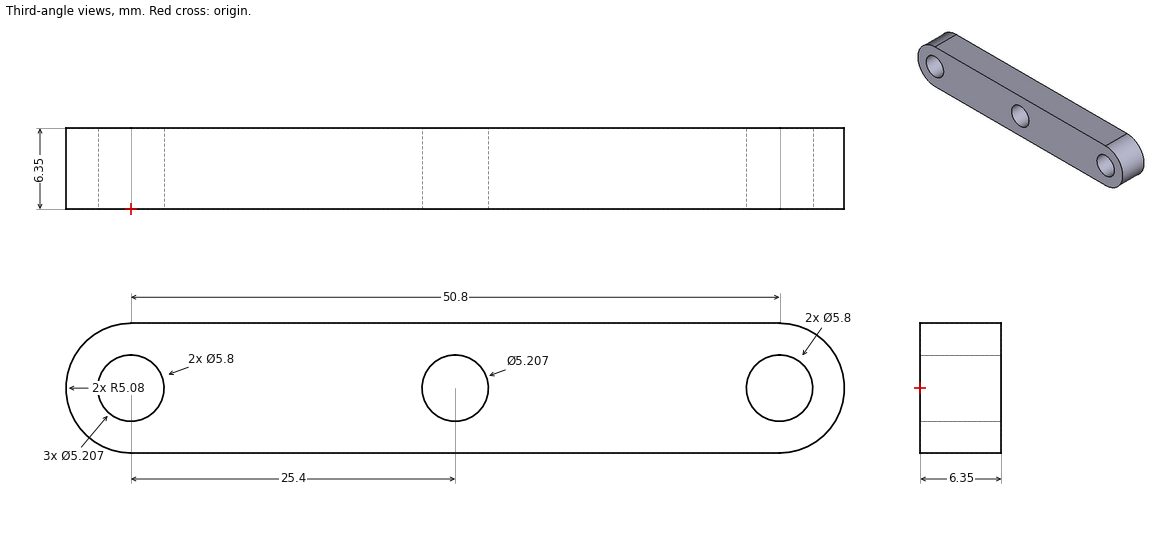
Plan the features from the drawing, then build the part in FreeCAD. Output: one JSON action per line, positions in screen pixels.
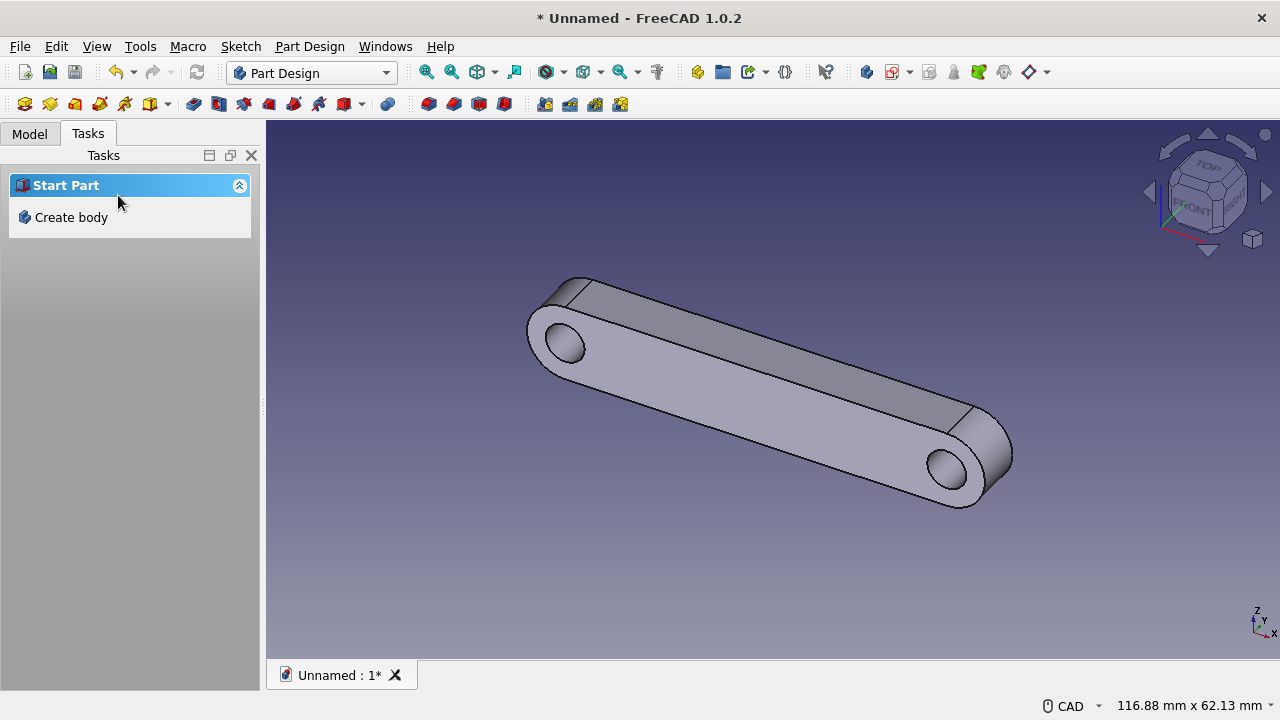
{"action": "key", "text": "4"}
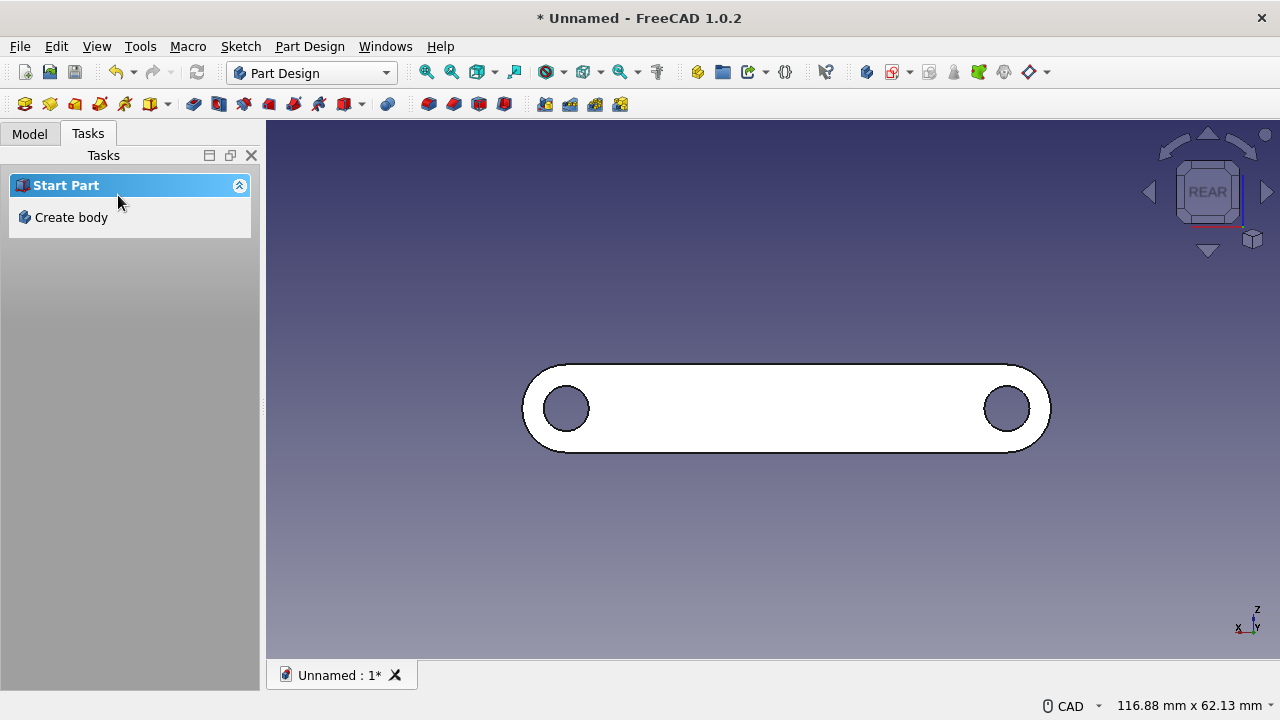
{"action": "left_click", "coordinate": [635, 408]}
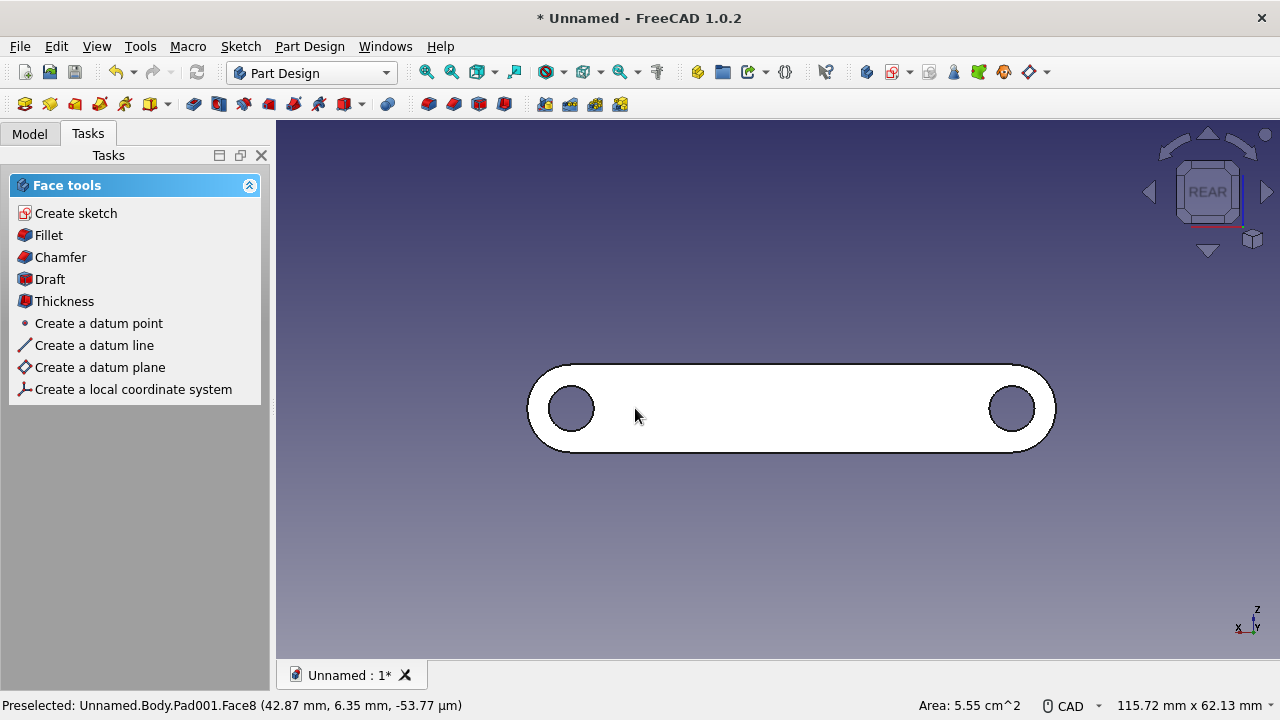
{"action": "left_click", "coordinate": [892, 72]}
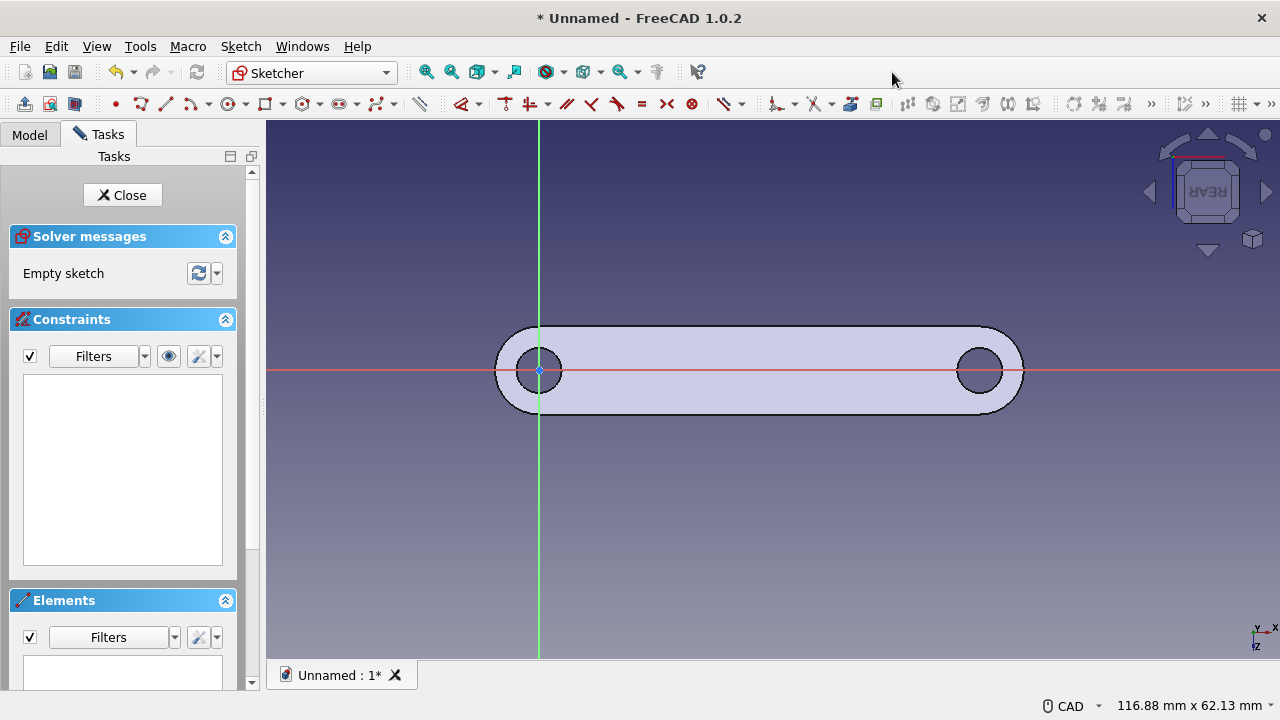
{"action": "scroll", "coordinate": [768, 367], "scroll_direction": "up", "scroll_amount": 10}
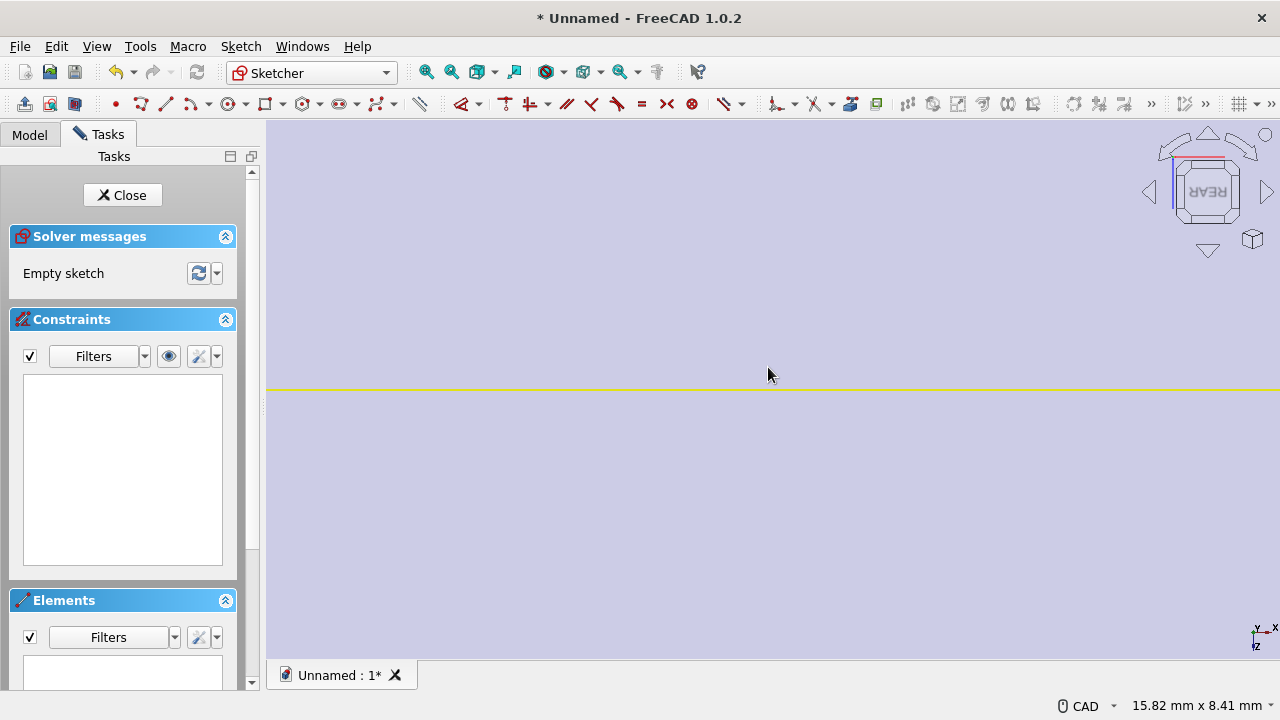
{"action": "left_click", "coordinate": [228, 104]}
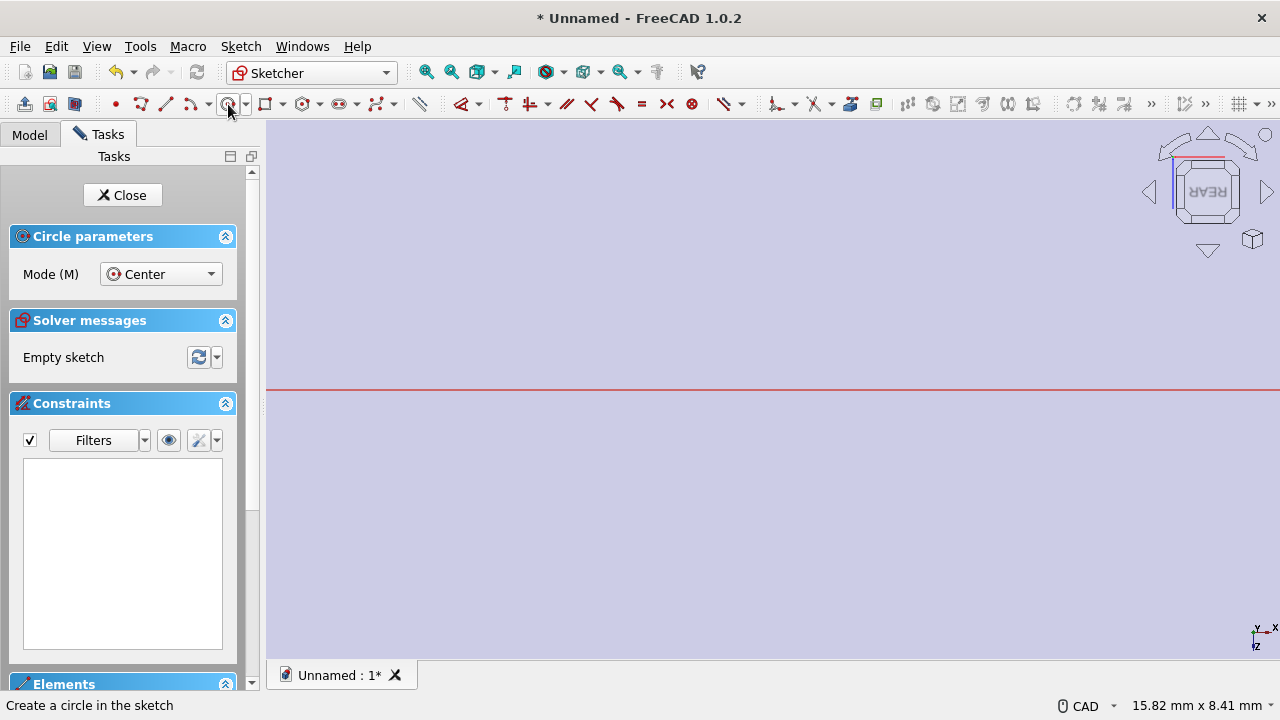
{"action": "left_click", "coordinate": [701, 390]}
{"action": "mouse_move", "coordinate": [819, 272]}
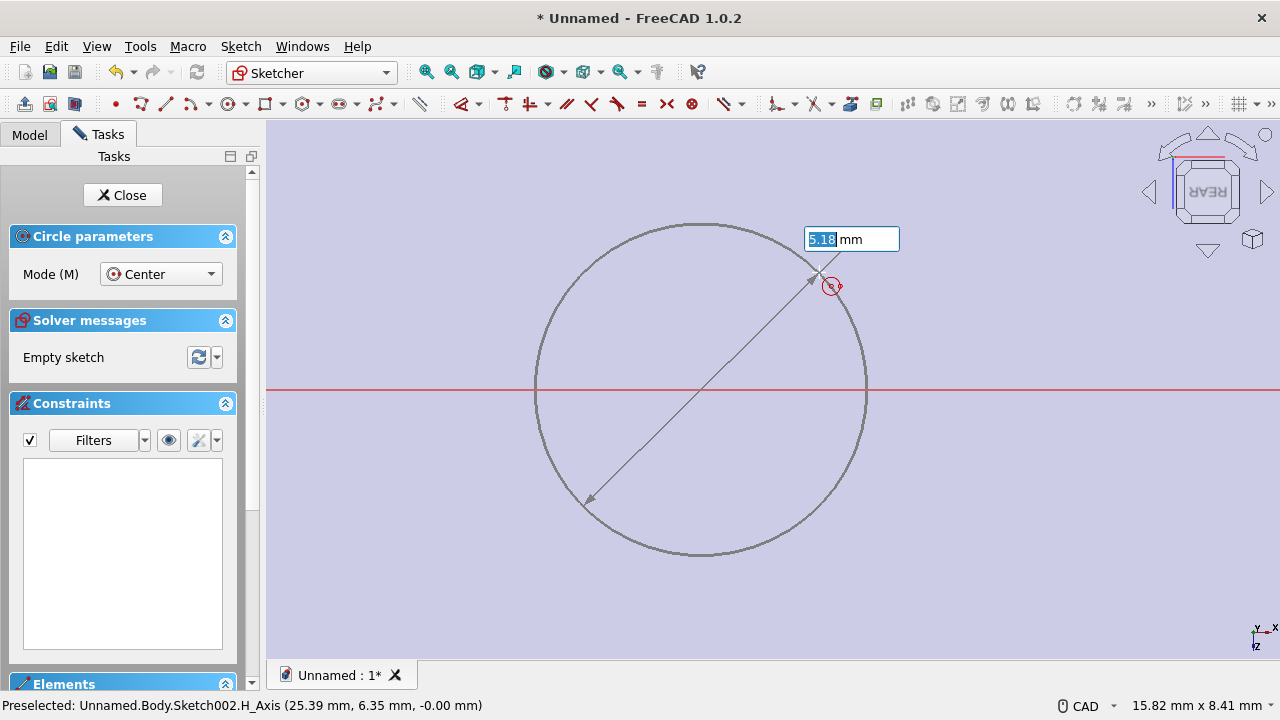
{"action": "type", "text": "5.207"}
{"action": "key", "text": "Return"}
{"action": "key", "text": "Escape"}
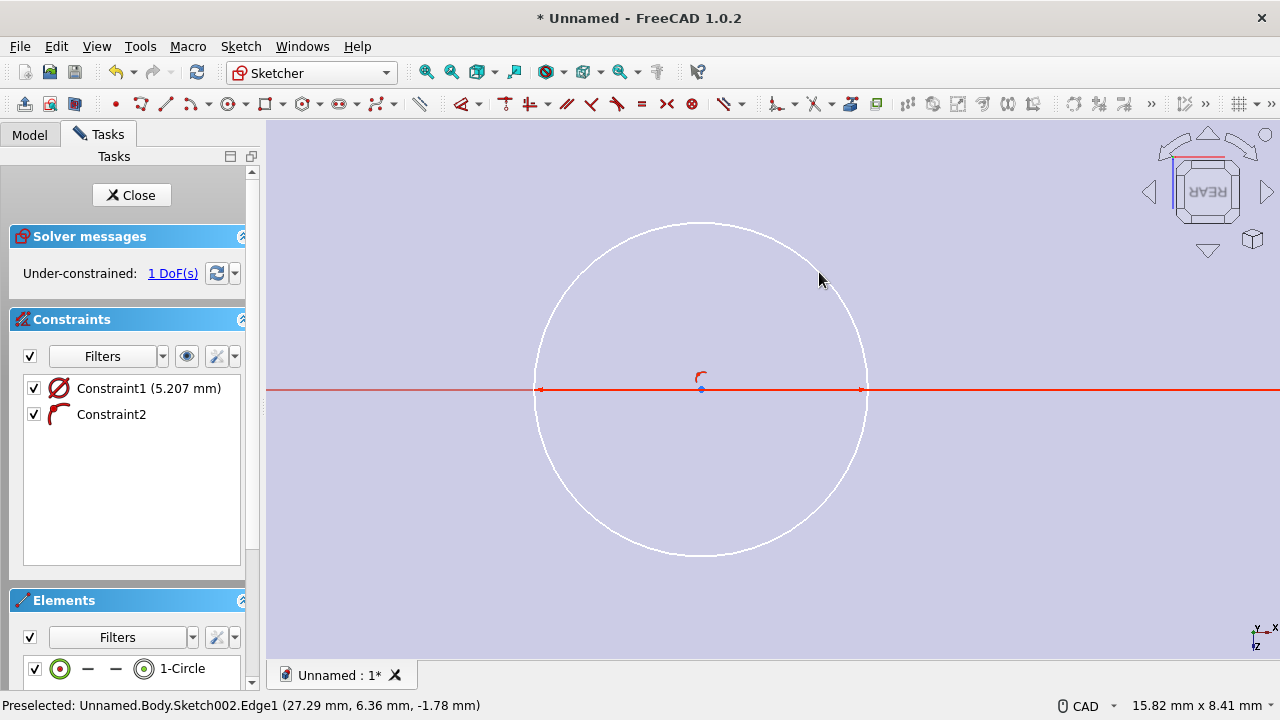
{"action": "key", "text": "d"}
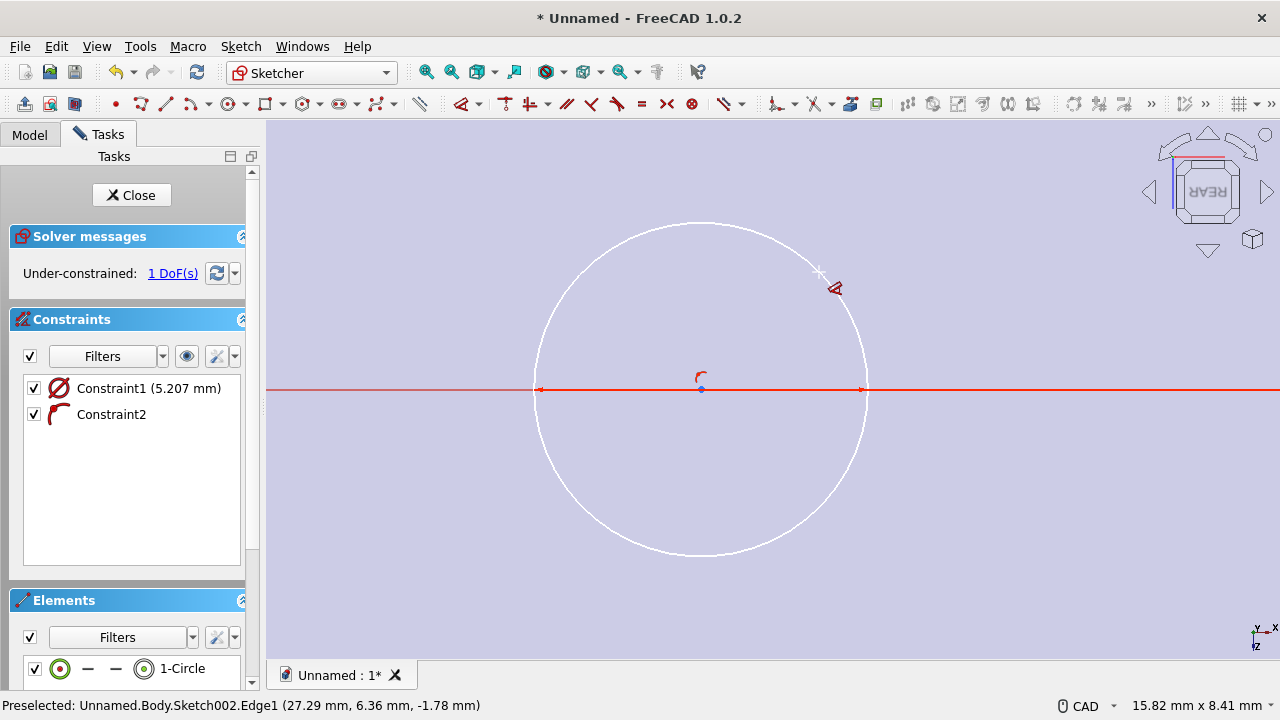
{"action": "left_click", "coordinate": [701, 390]}
{"action": "left_click", "coordinate": [498, 424]}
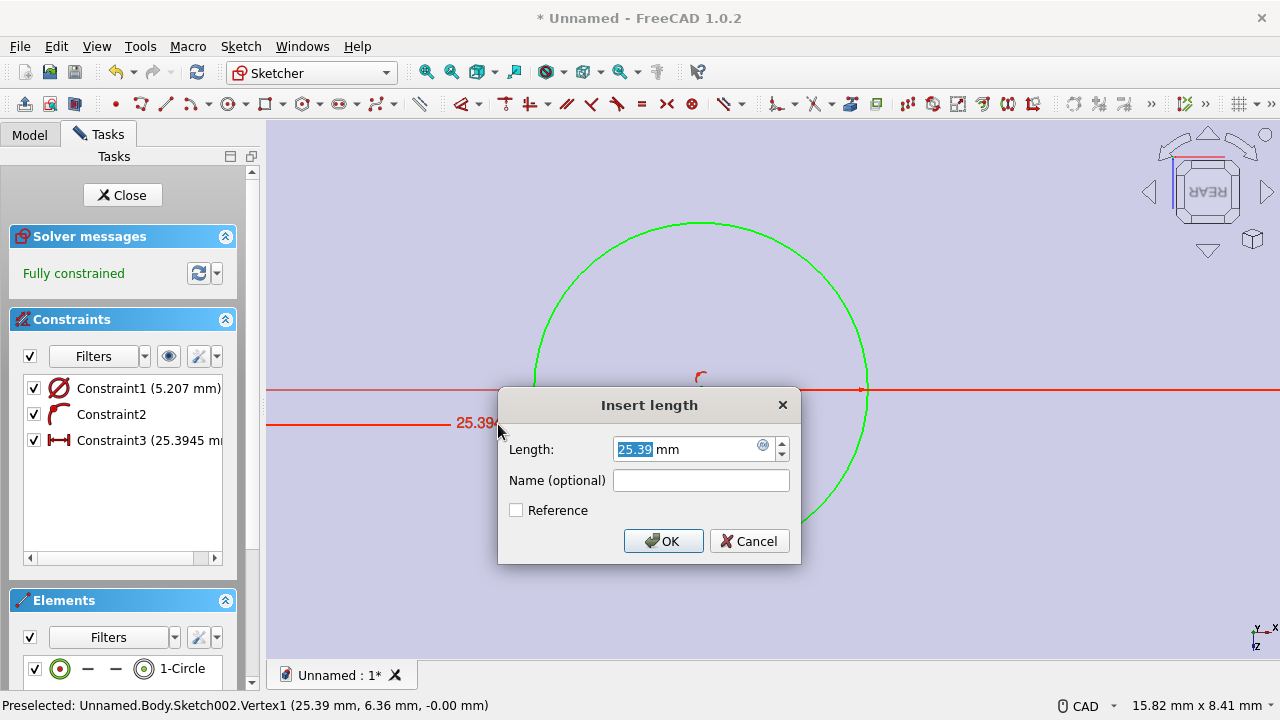
{"action": "type", "text": "25.4"}
{"action": "key", "text": "Return"}
{"action": "key", "text": "Escape"}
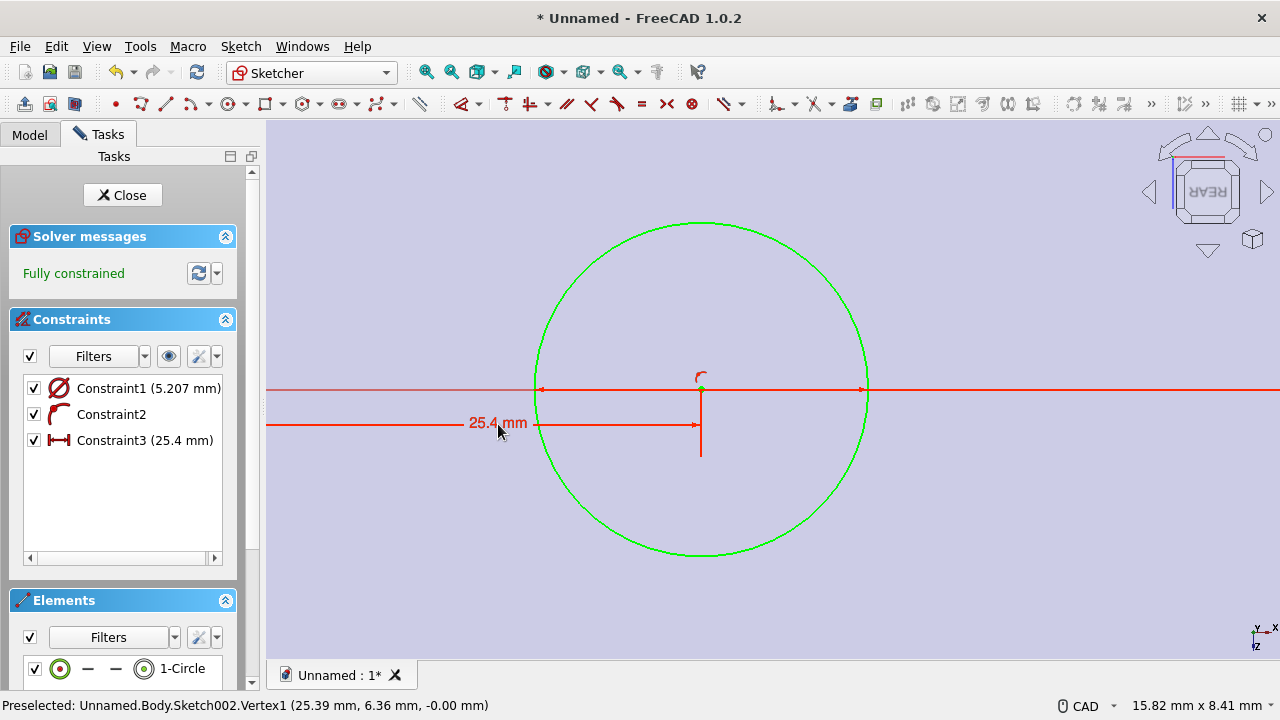
{"action": "left_click", "coordinate": [123, 195]}